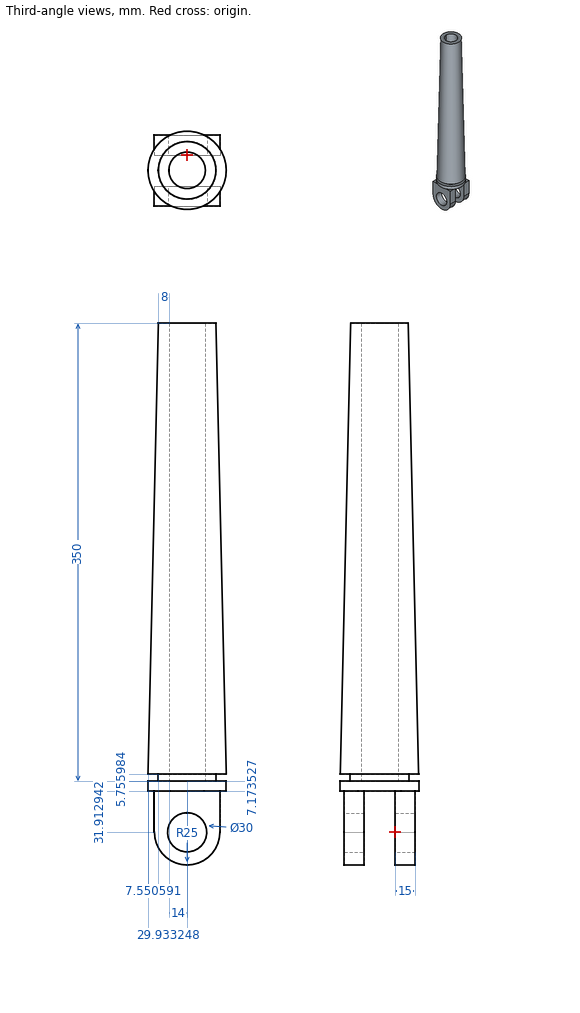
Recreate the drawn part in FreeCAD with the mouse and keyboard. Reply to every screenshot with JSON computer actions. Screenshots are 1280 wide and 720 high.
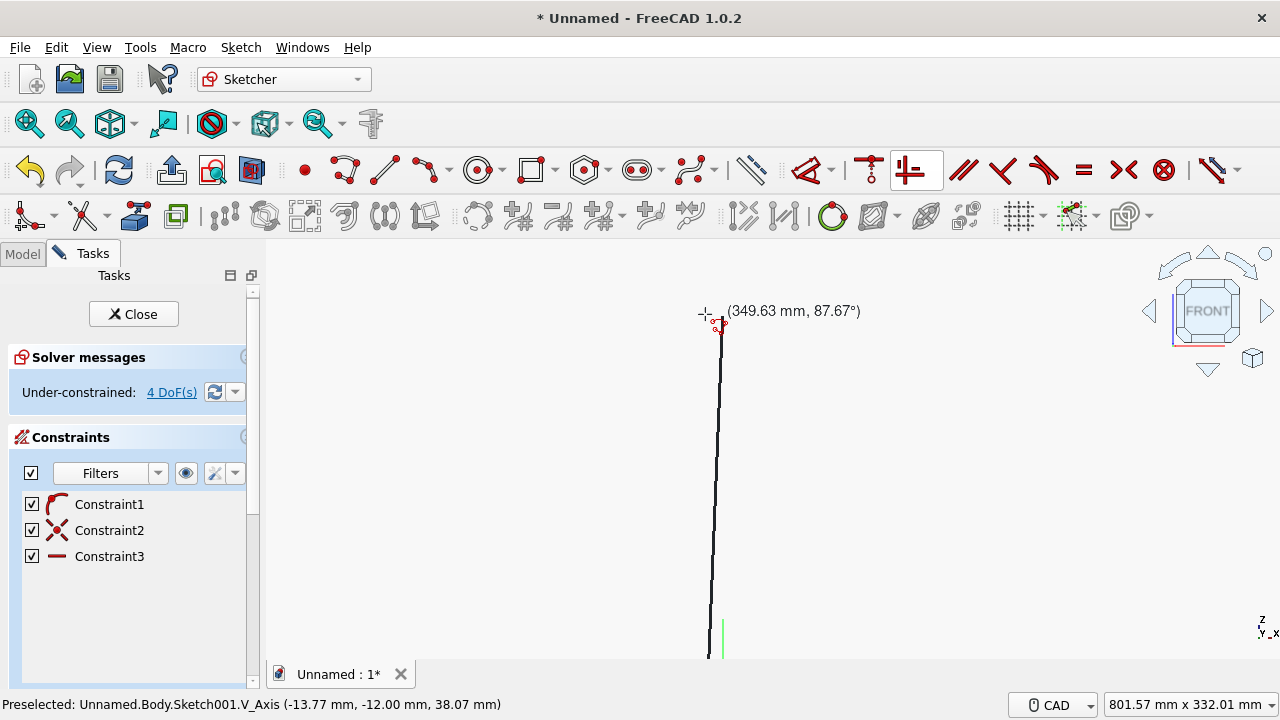
{"action": "left_click", "coordinate": [705, 314]}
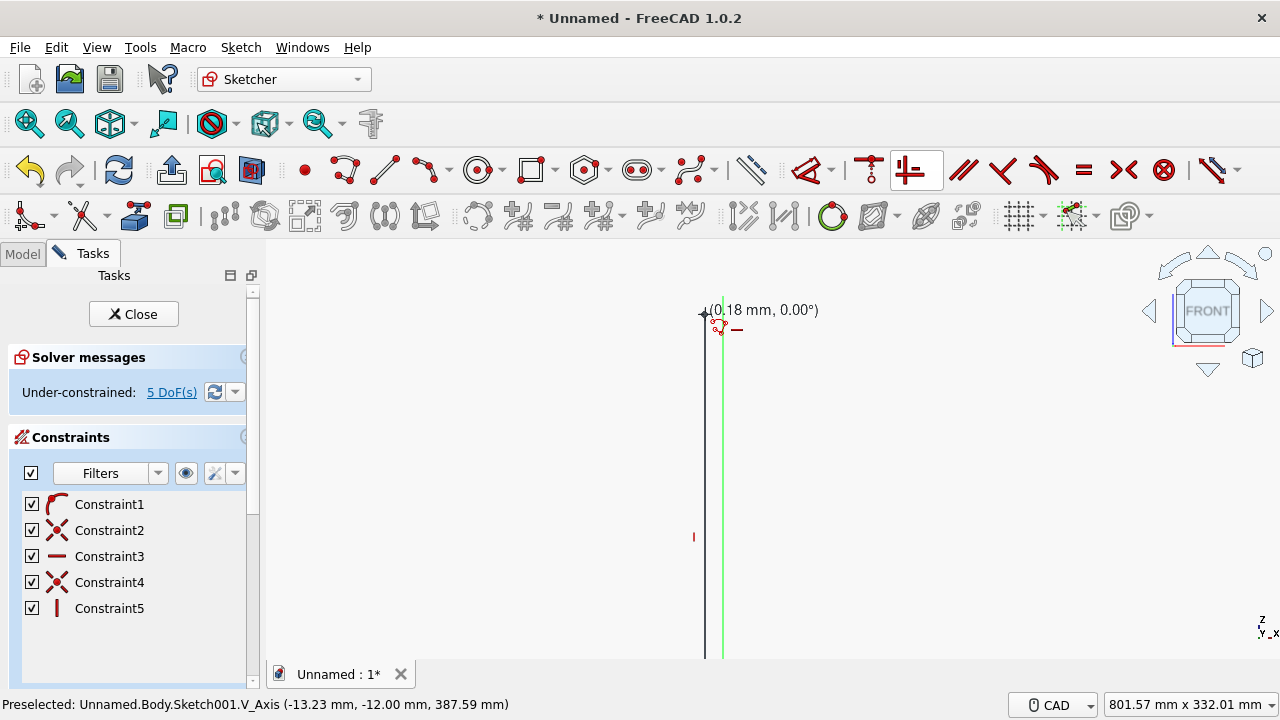
{"action": "scroll", "coordinate": [695, 314], "scroll_direction": "up", "scroll_amount": 3}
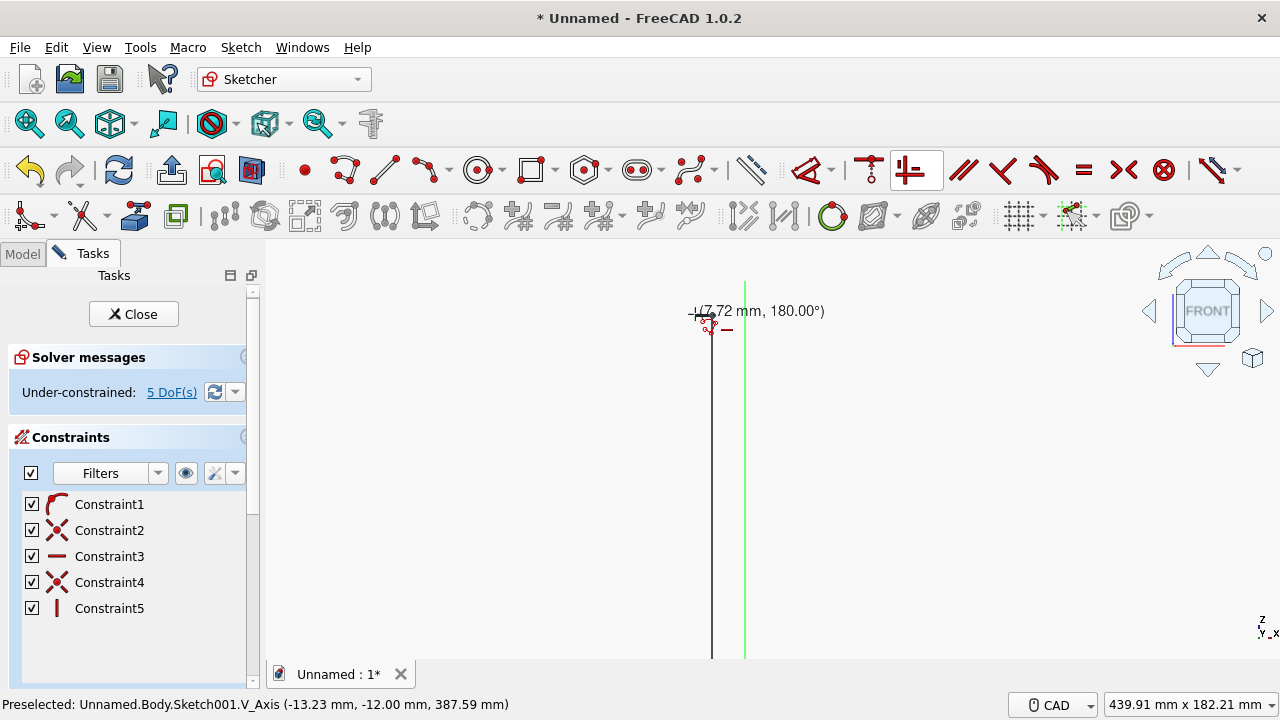
{"action": "left_click", "coordinate": [694, 314]}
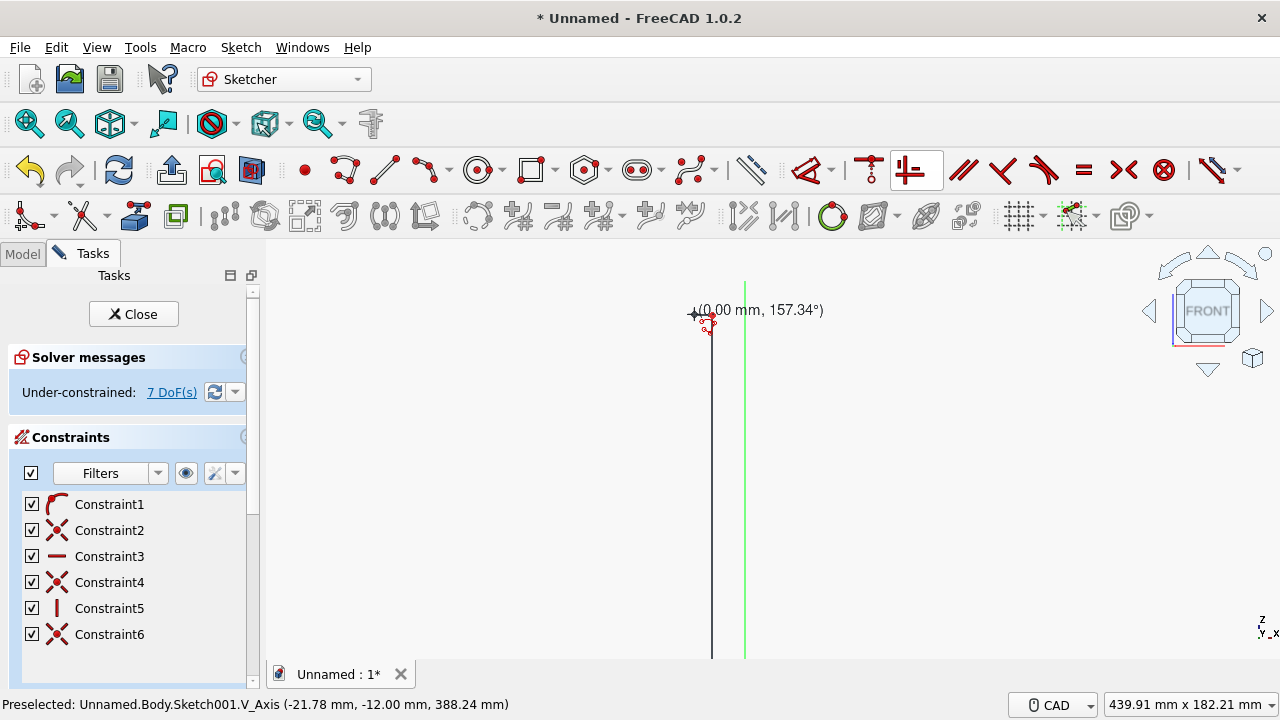
{"action": "scroll", "coordinate": [702, 314], "scroll_direction": "down", "scroll_amount": 6}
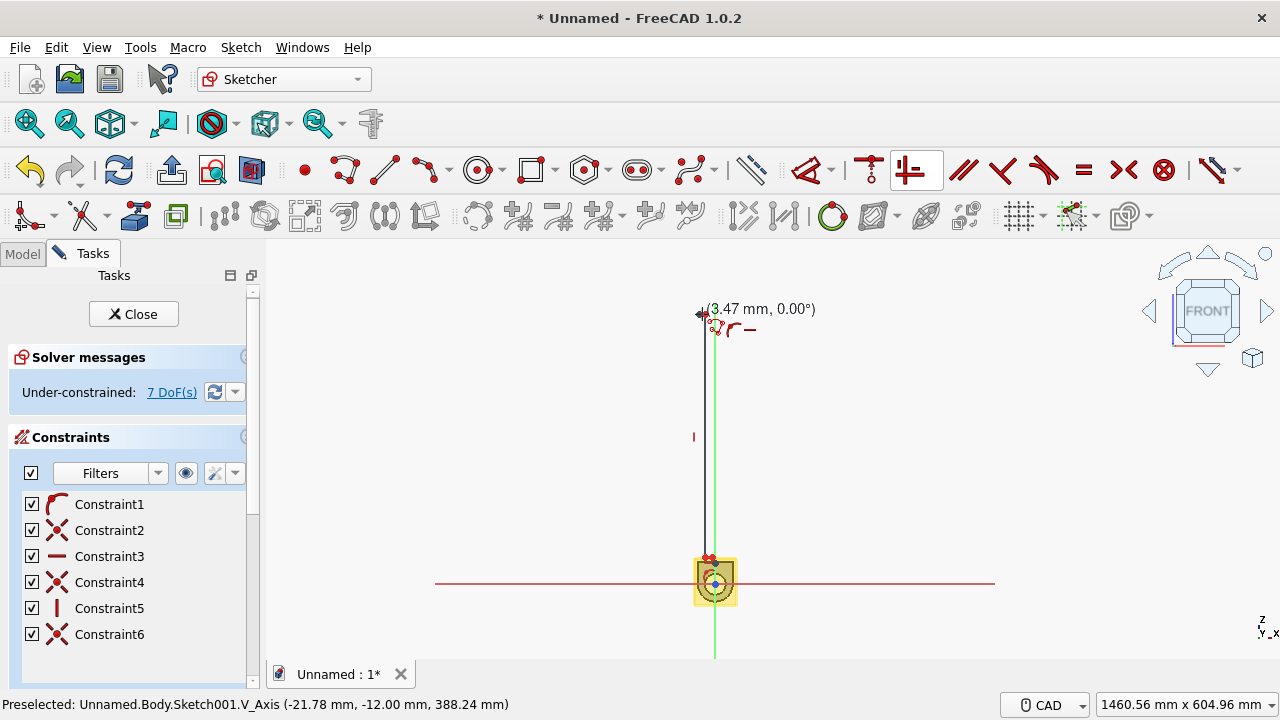
{"action": "scroll", "coordinate": [695, 553], "scroll_direction": "up", "scroll_amount": 2}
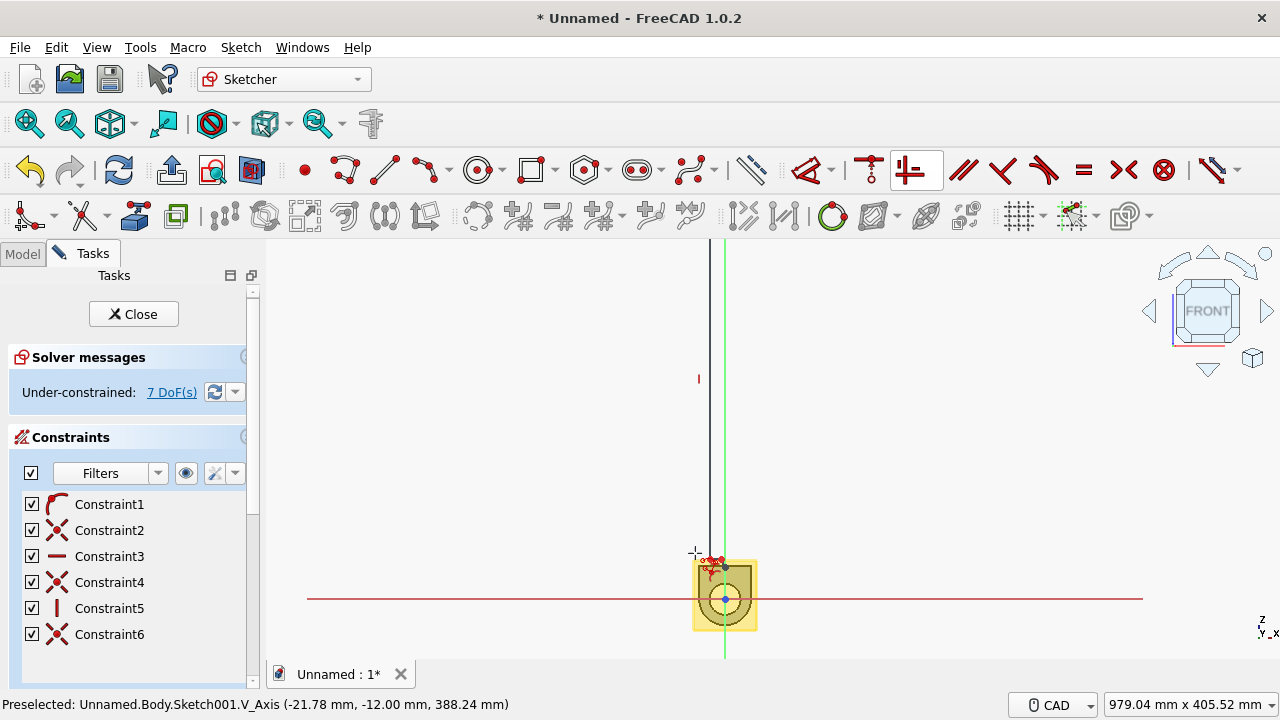
{"action": "left_click", "coordinate": [685, 553]}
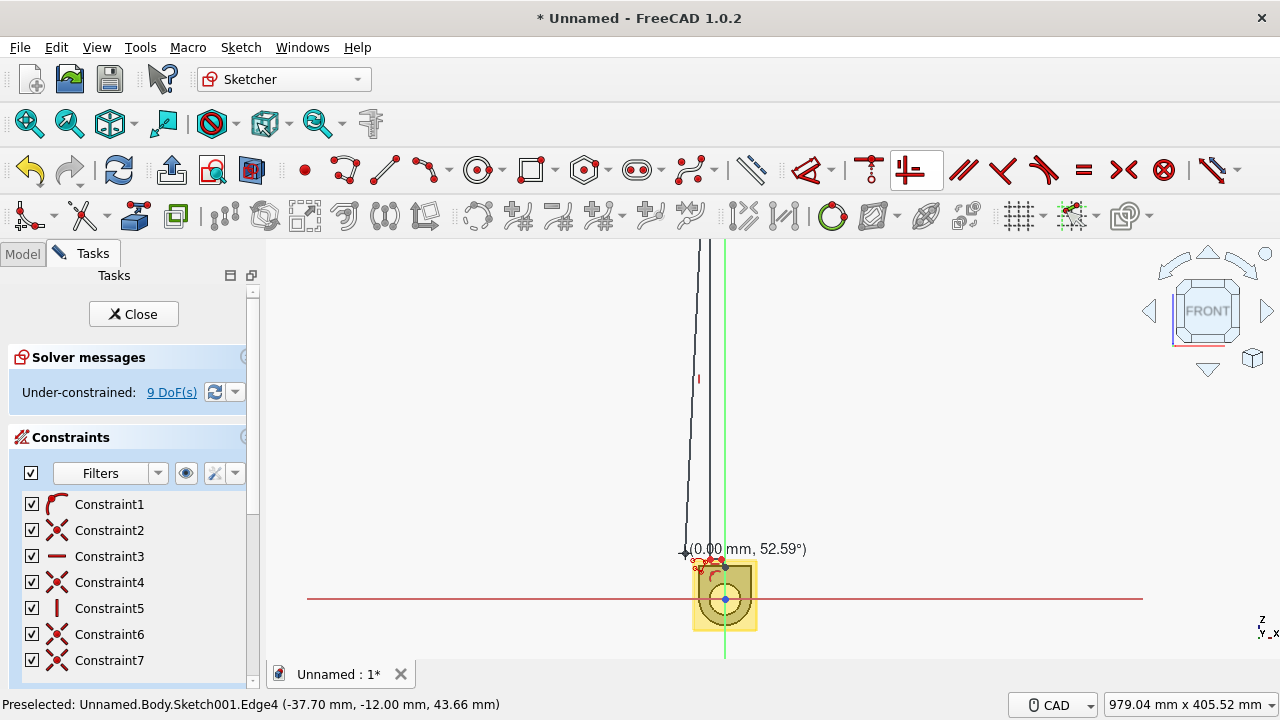
{"action": "scroll", "coordinate": [702, 553], "scroll_direction": "up", "scroll_amount": 4}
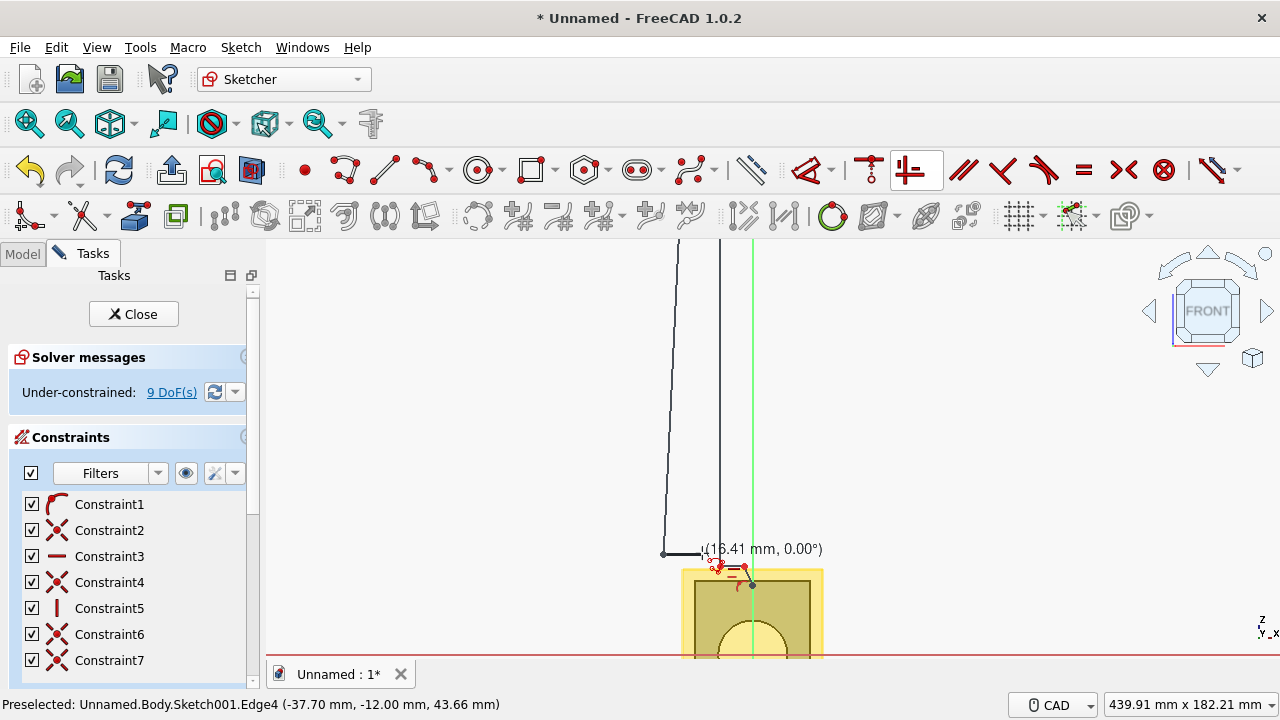
{"action": "left_click", "coordinate": [701, 552]}
{"action": "left_click", "coordinate": [701, 565]}
{"action": "left_click", "coordinate": [684, 565]}
{"action": "left_click", "coordinate": [684, 581]}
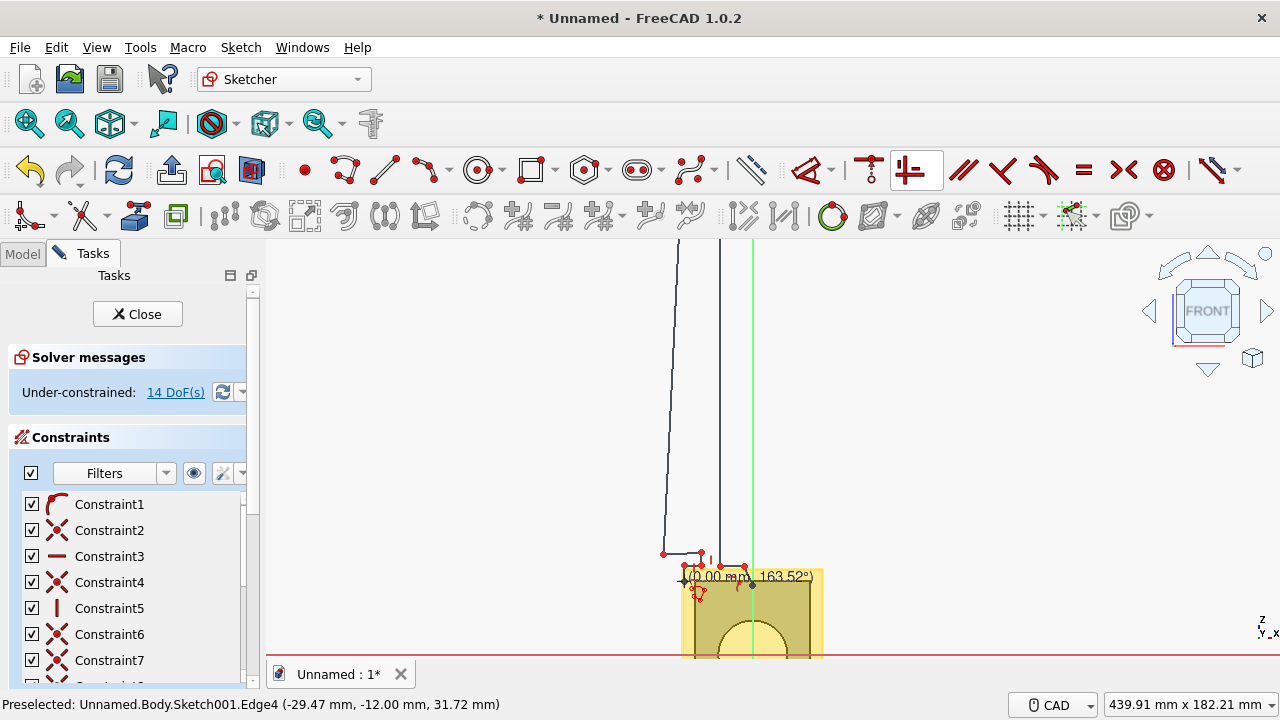
{"action": "scroll", "coordinate": [753, 581], "scroll_direction": "up", "scroll_amount": 4}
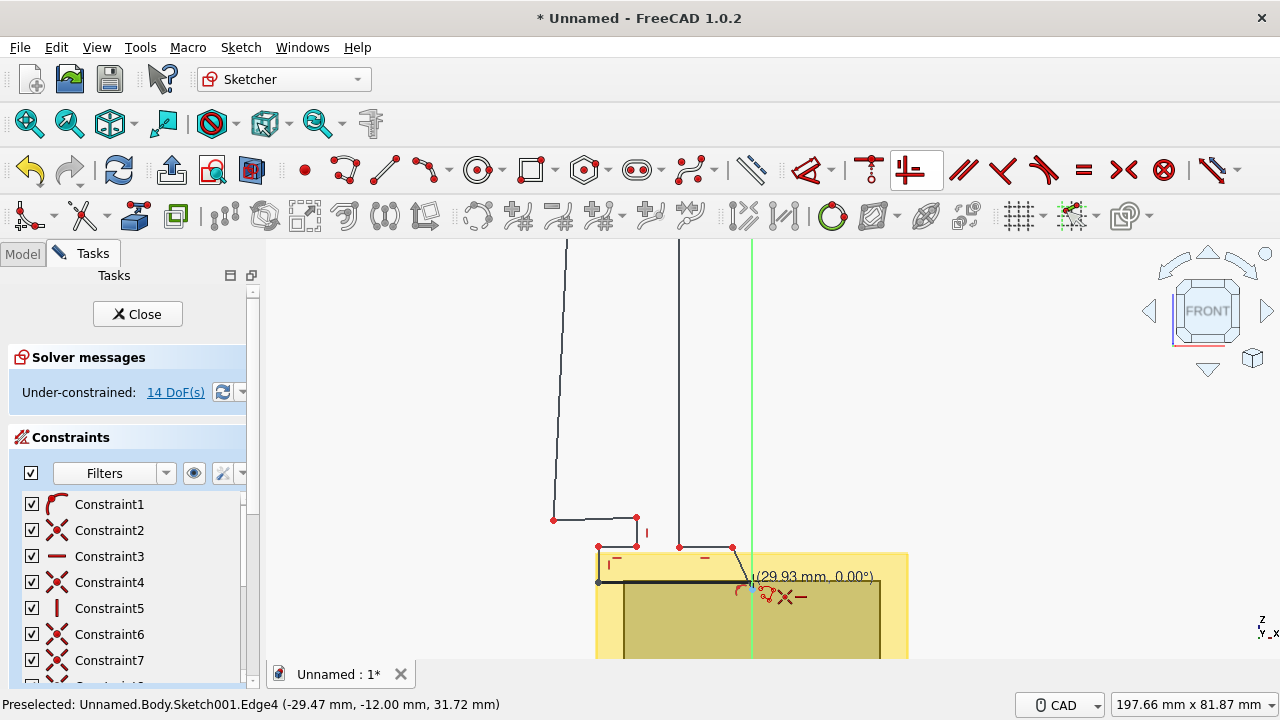
{"action": "left_click", "coordinate": [752, 590]}
{"action": "key", "text": "Escape"}
{"action": "key", "text": "Escape"}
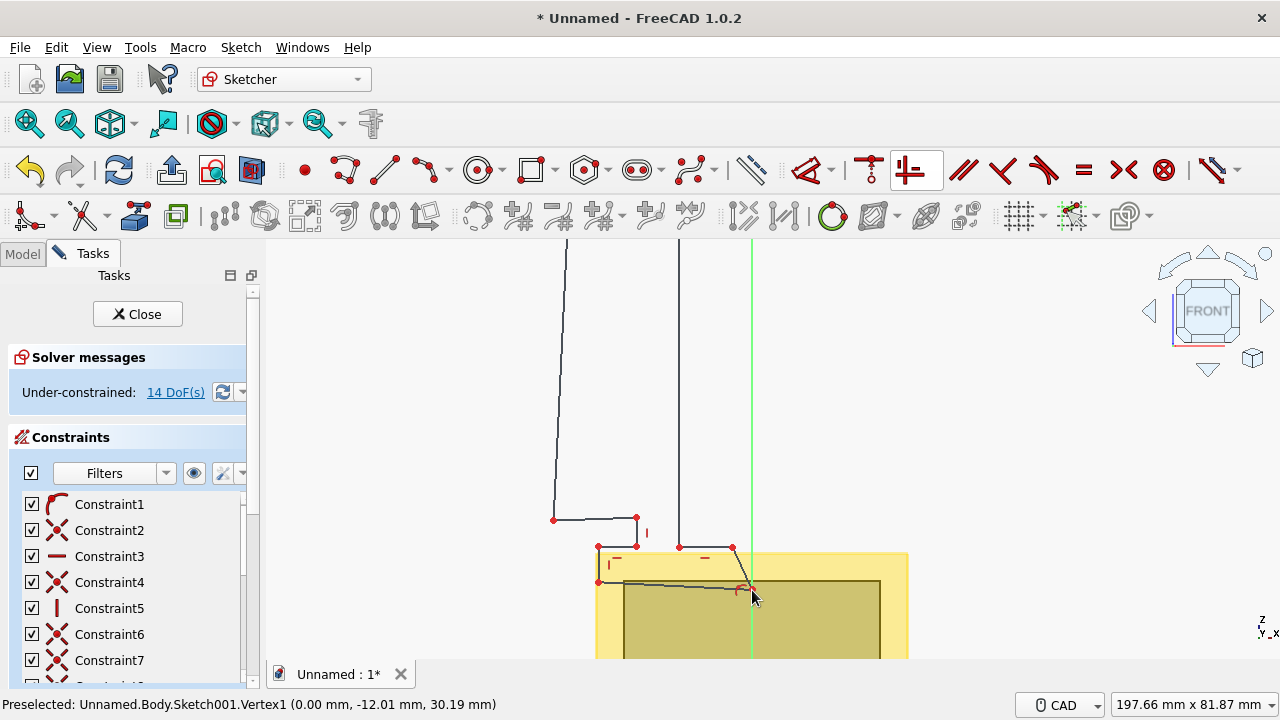
{"action": "left_click", "coordinate": [738, 560]}